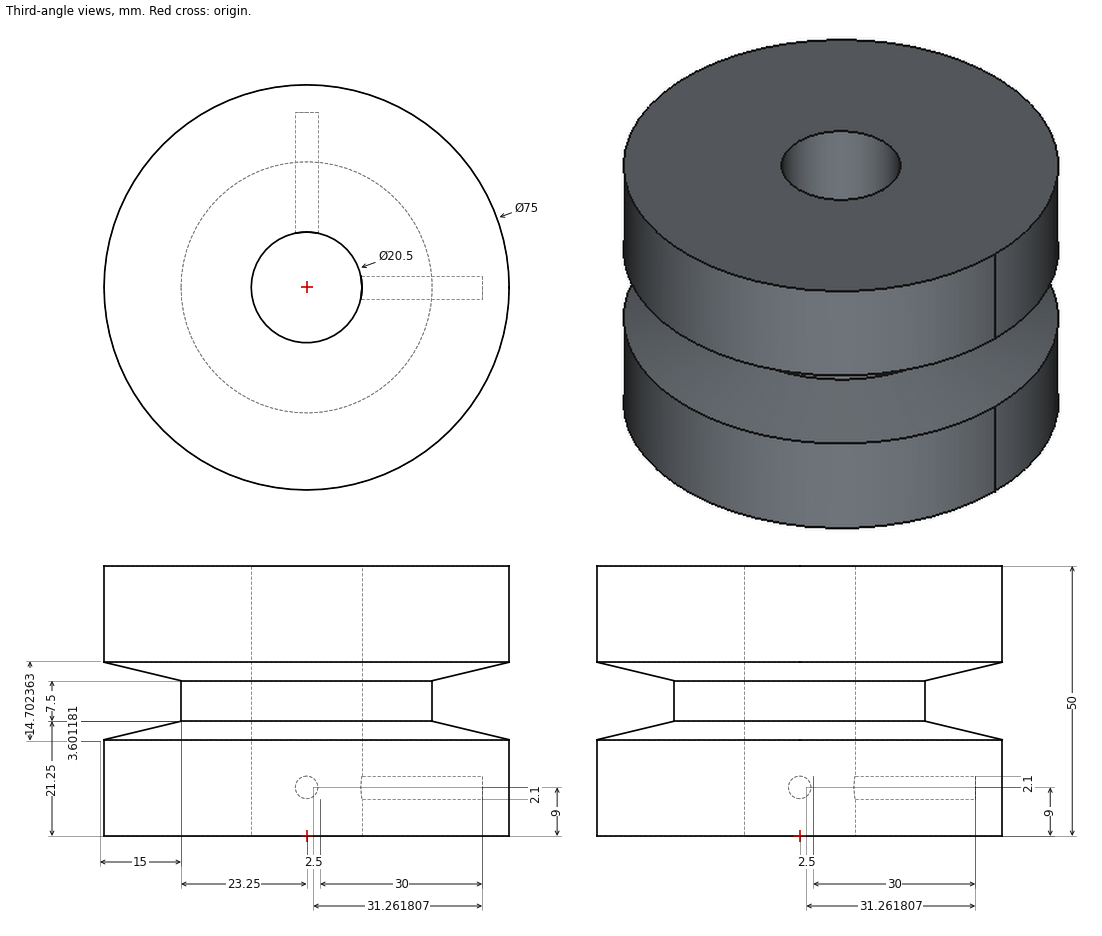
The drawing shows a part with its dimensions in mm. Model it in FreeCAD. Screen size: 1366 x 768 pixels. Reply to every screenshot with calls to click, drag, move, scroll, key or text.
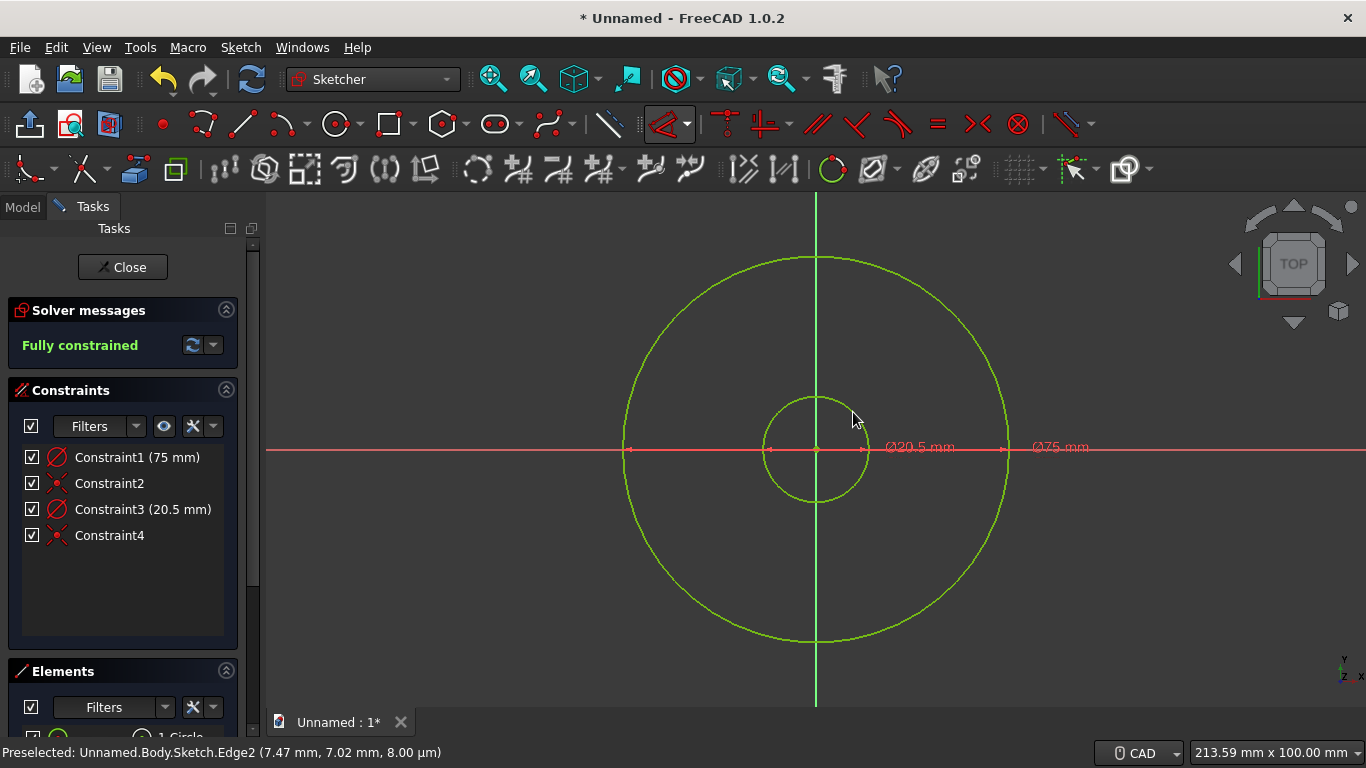
click(123, 267)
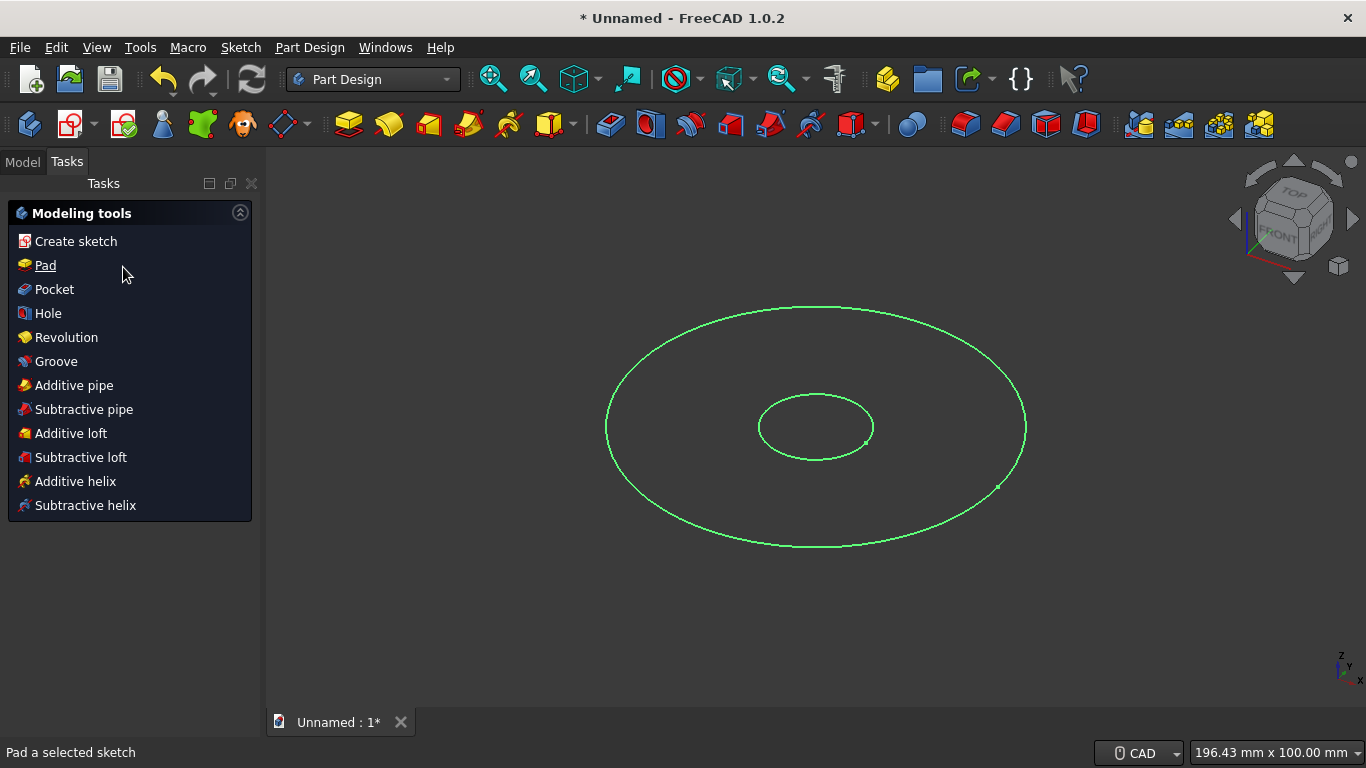
click(350, 124)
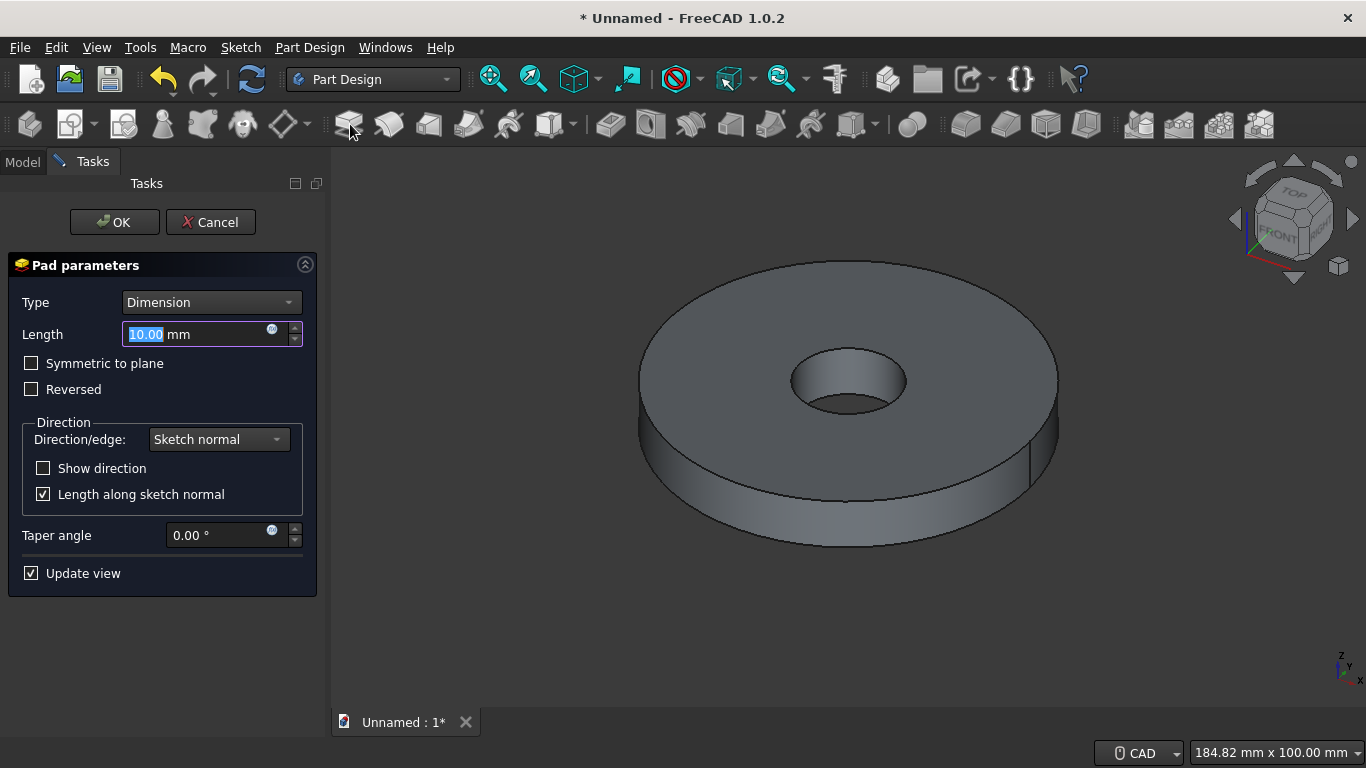
text(50)
key(Tab)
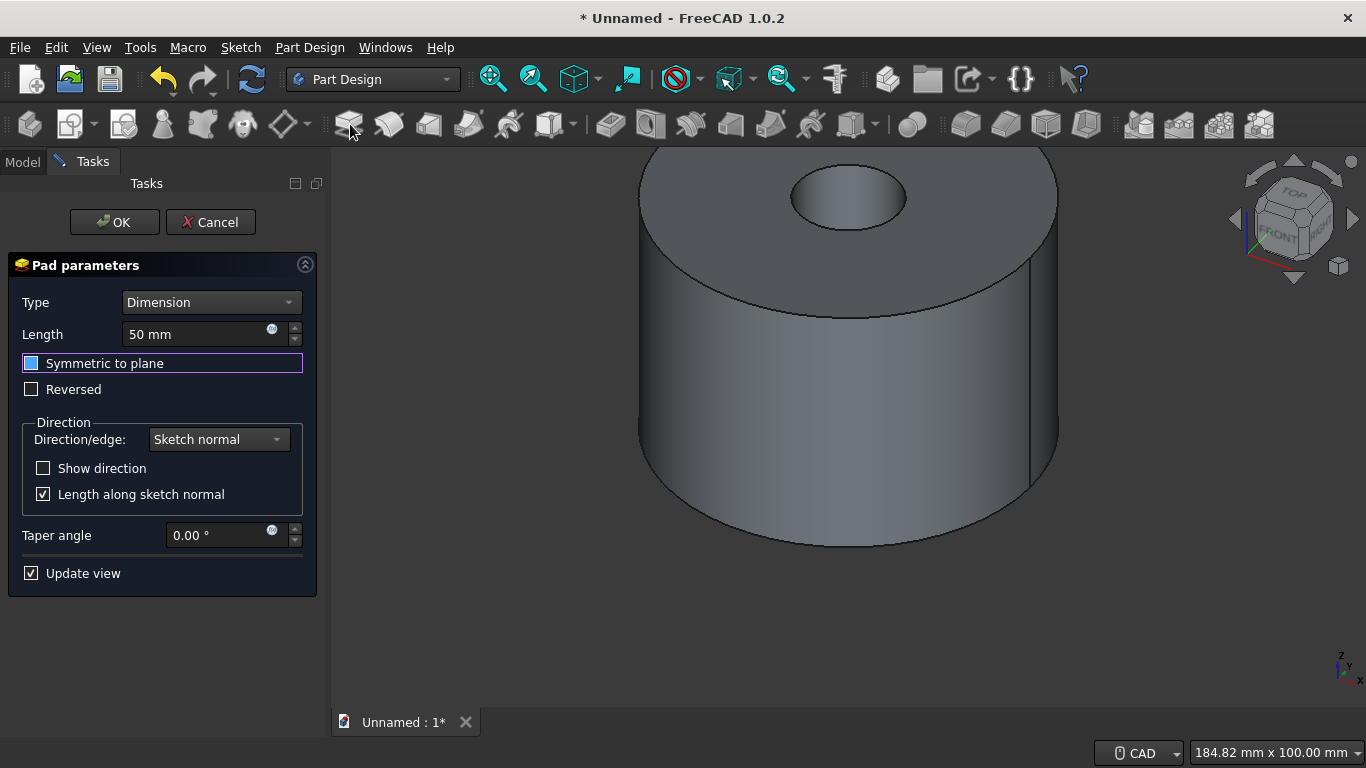
click(115, 222)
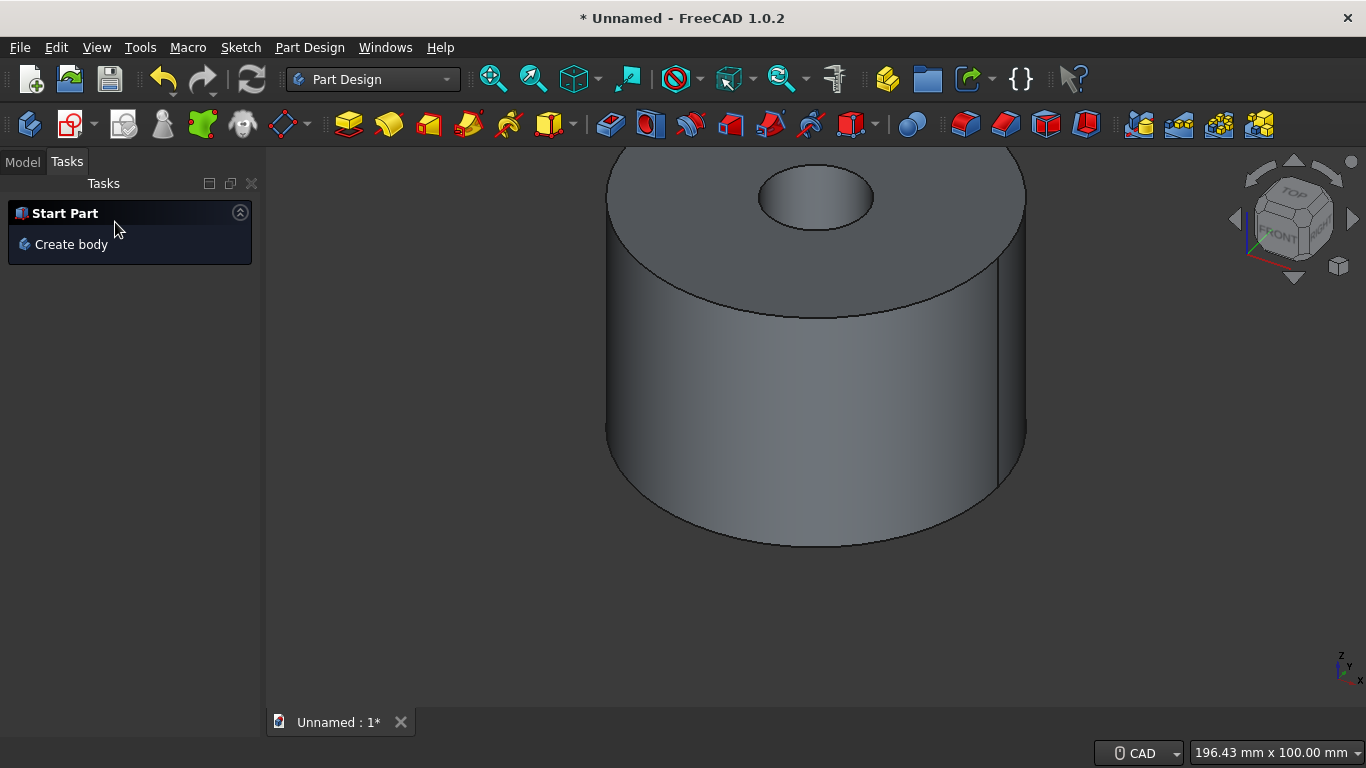
key(v)
key(f)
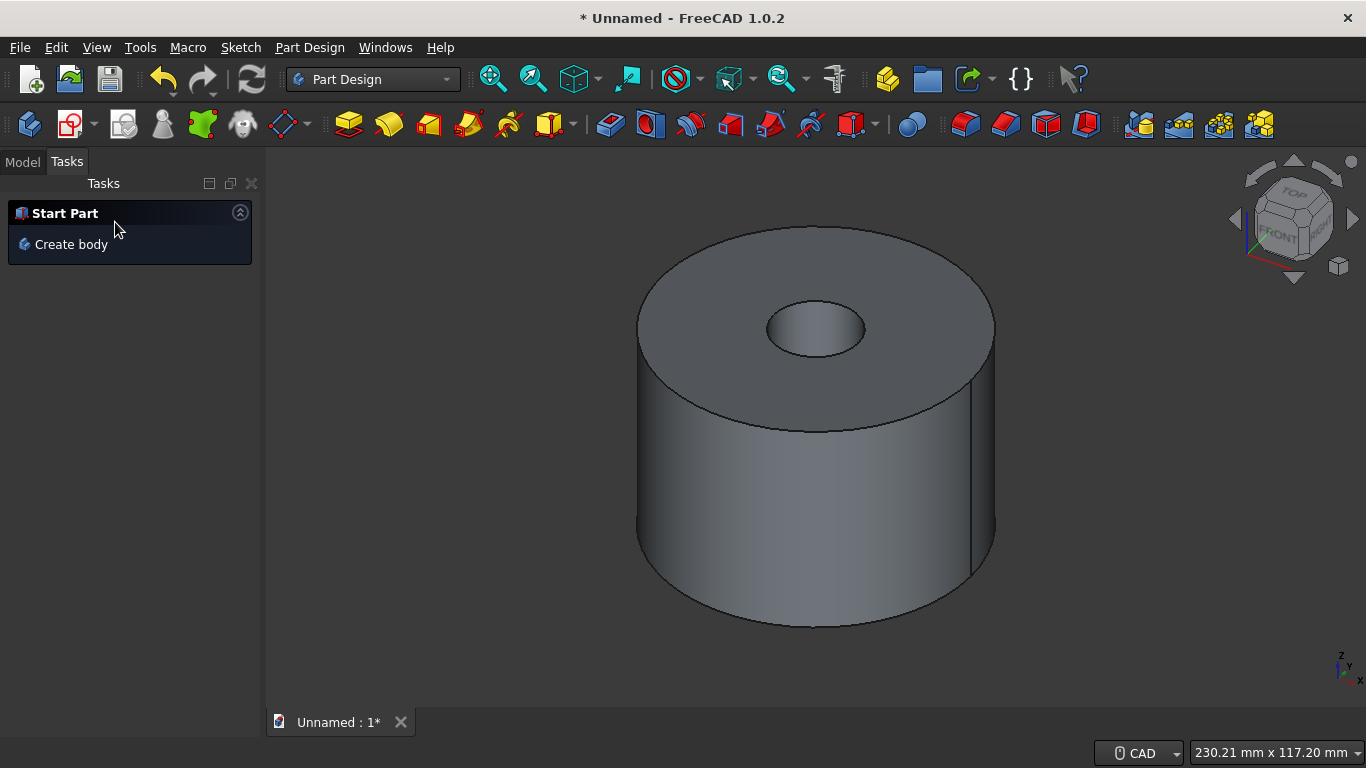
click(70, 124)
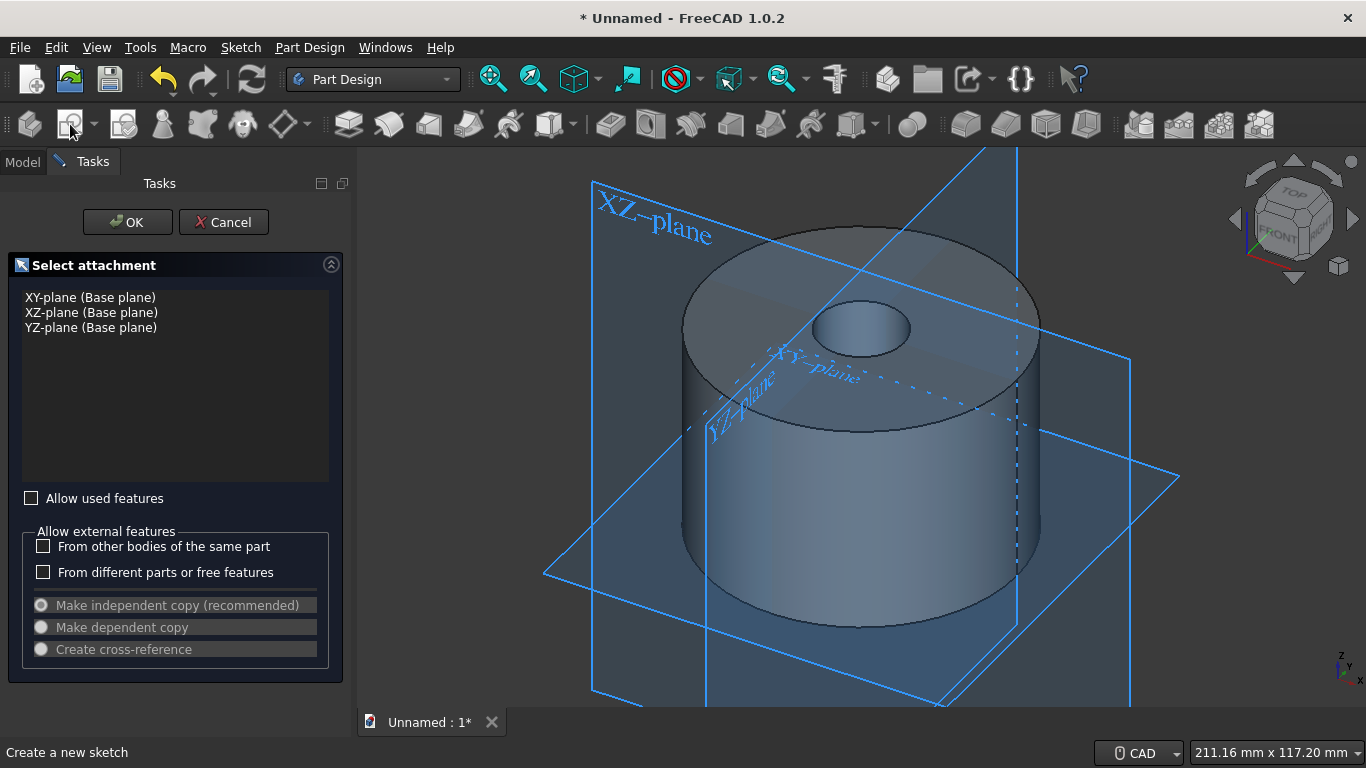
click(82, 312)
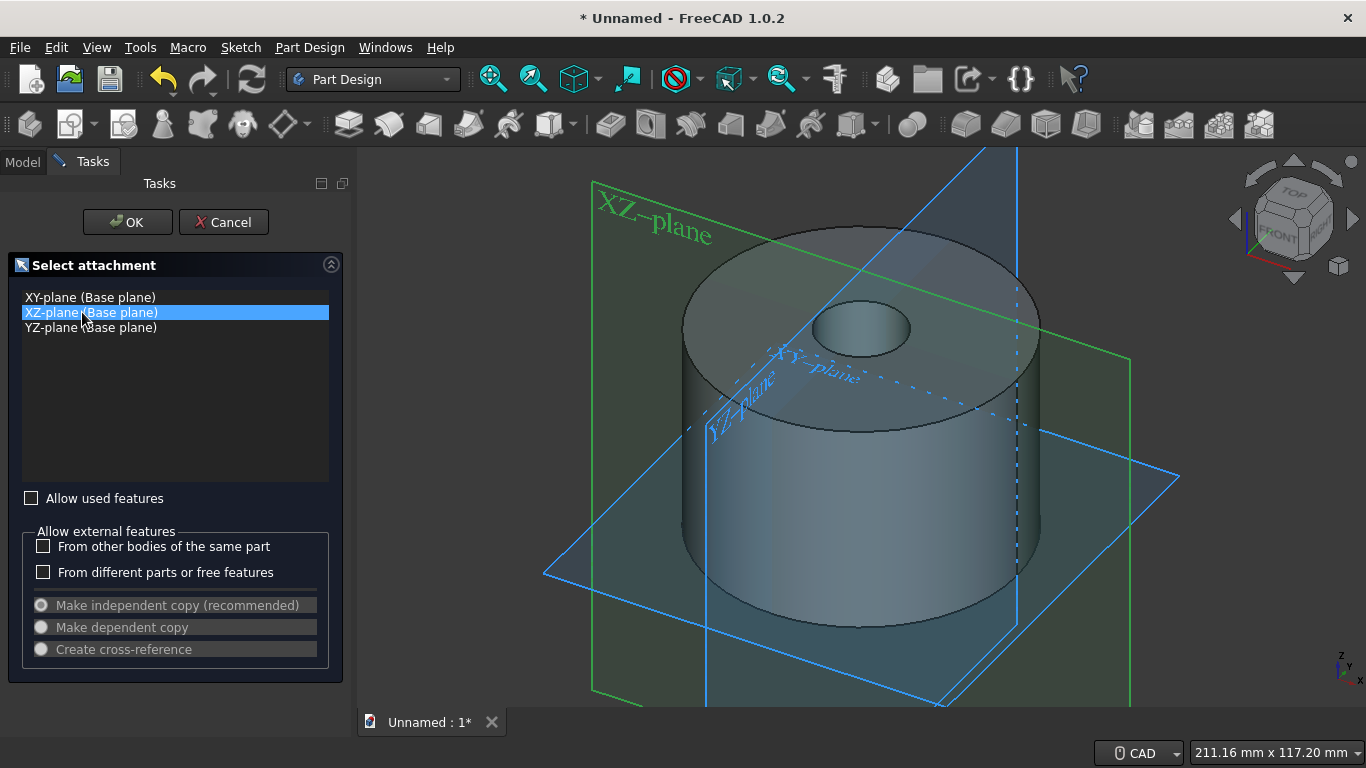
click(128, 222)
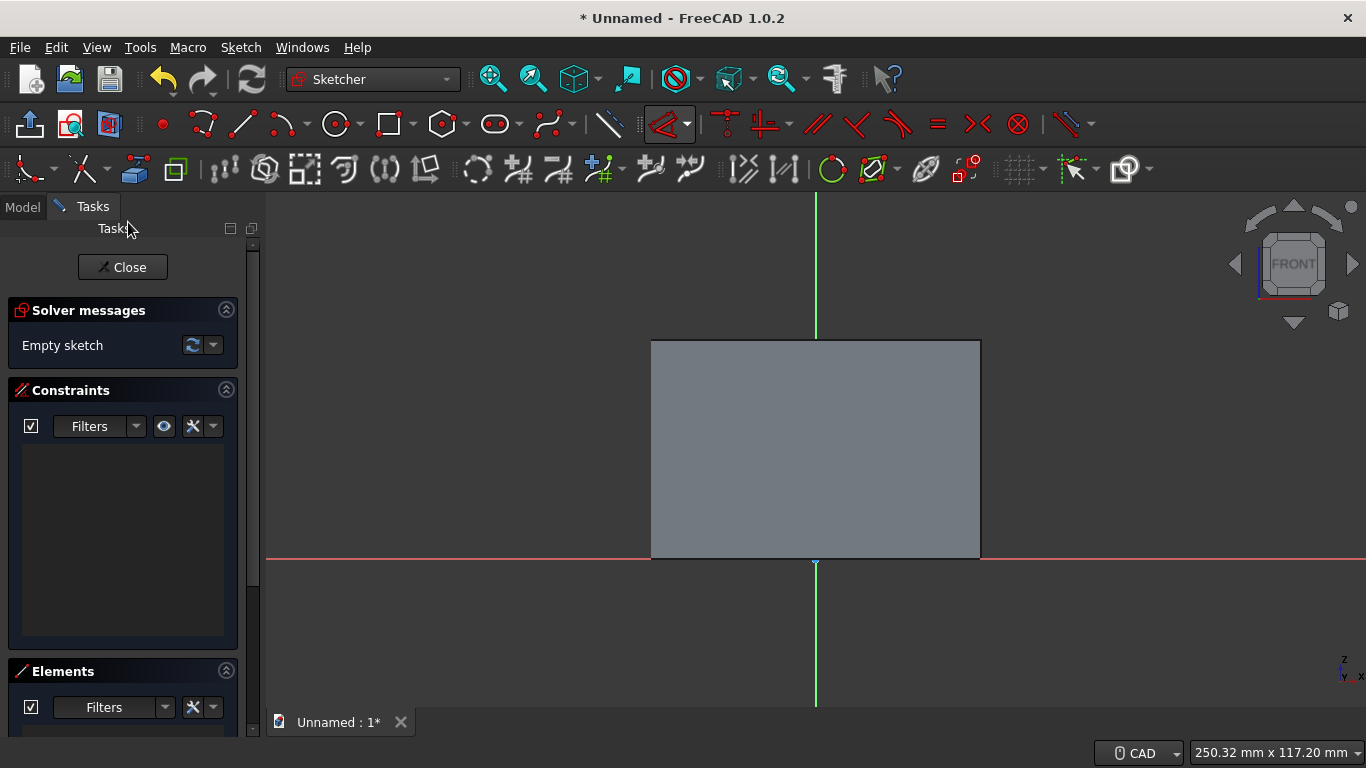
key(q)
key(s)